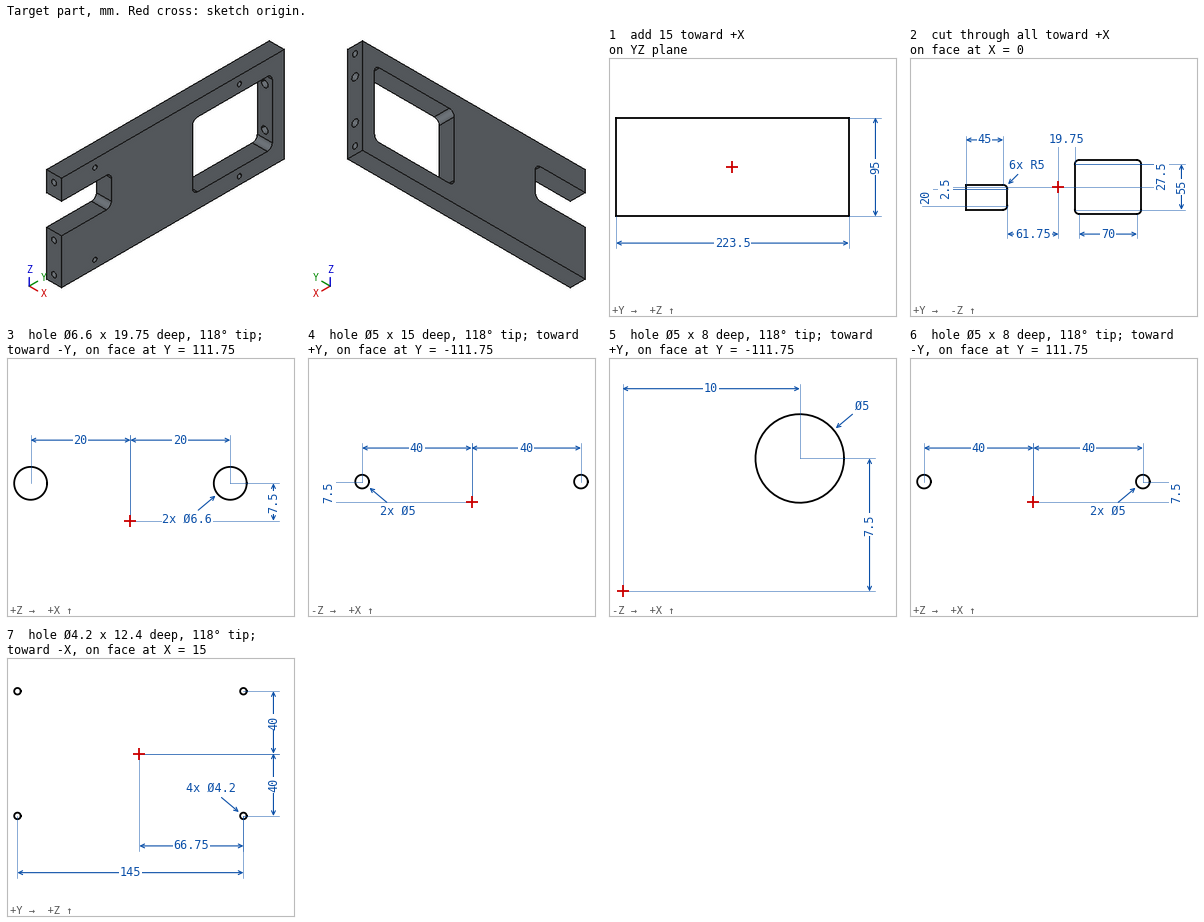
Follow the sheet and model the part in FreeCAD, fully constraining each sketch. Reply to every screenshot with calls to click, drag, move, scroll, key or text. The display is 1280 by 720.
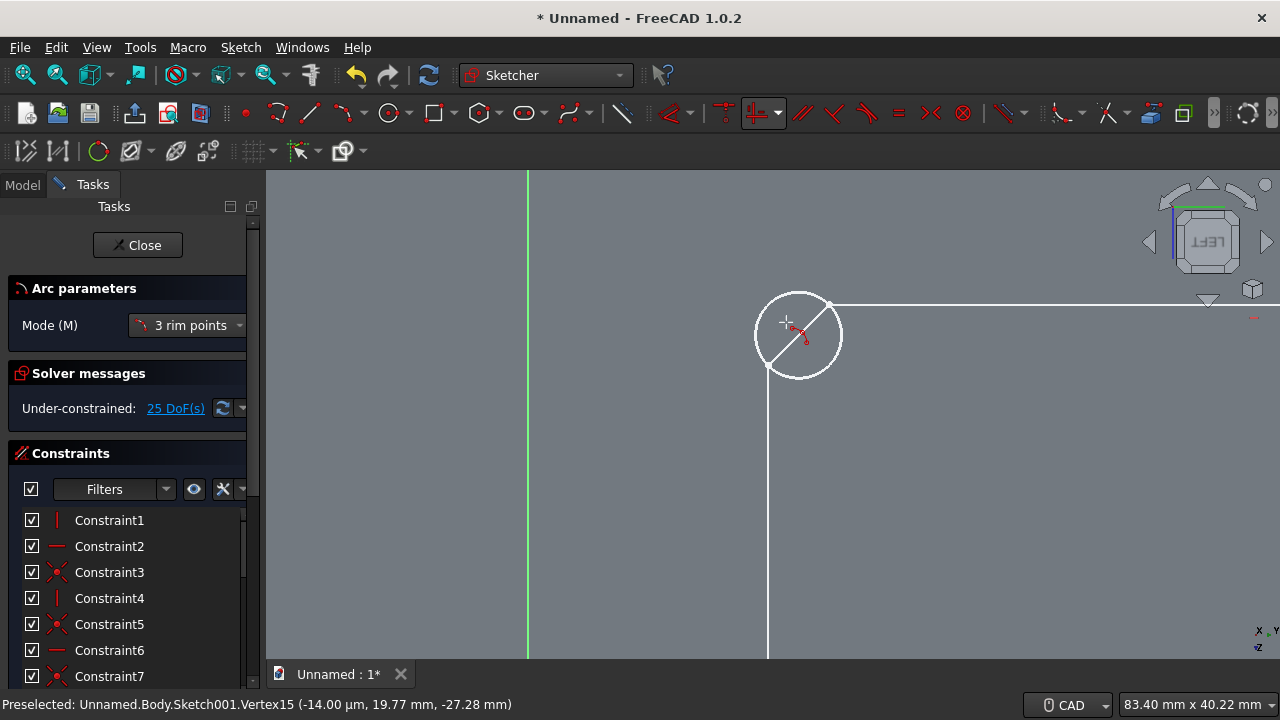
click(786, 320)
key(Escape)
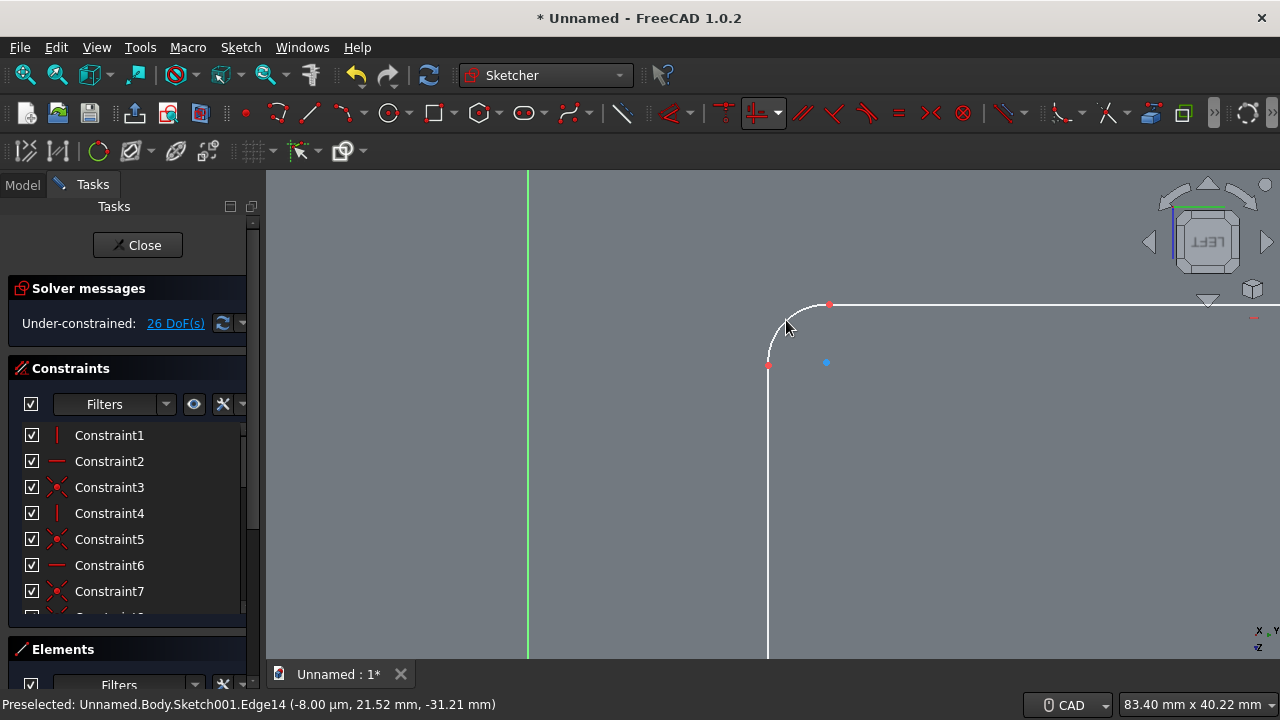
scroll(786, 322, down, 7)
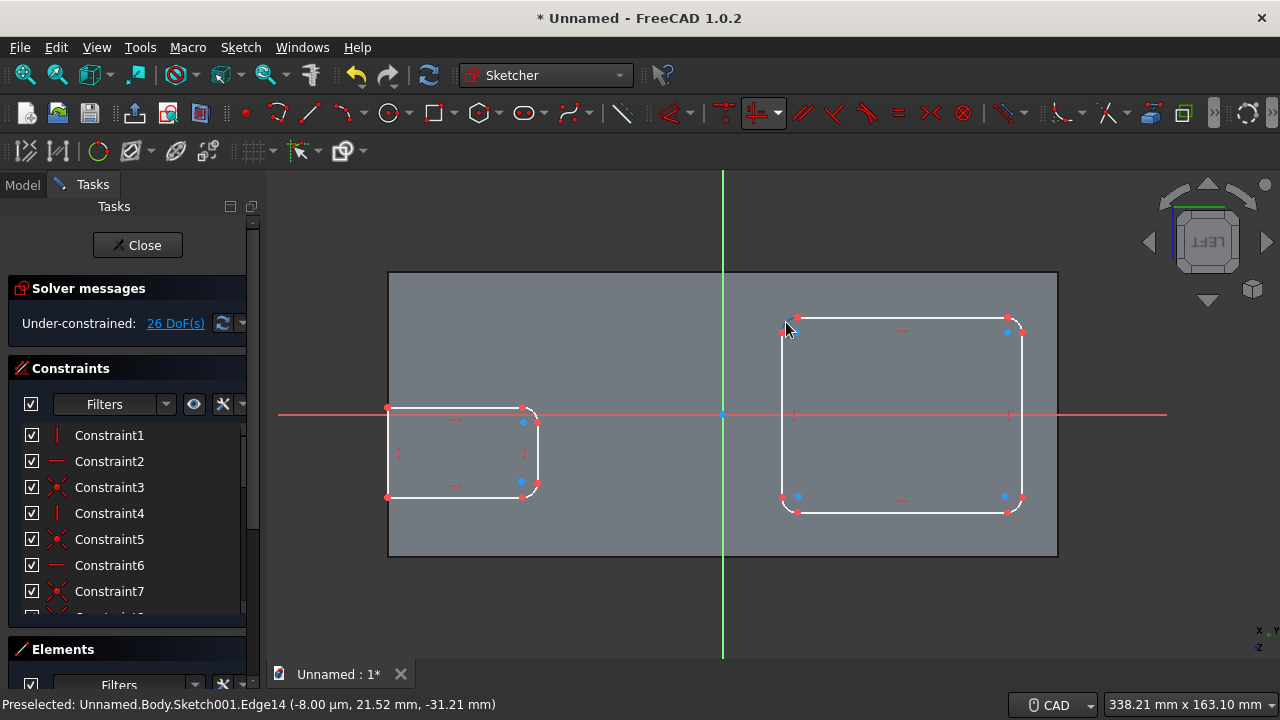
click(538, 465)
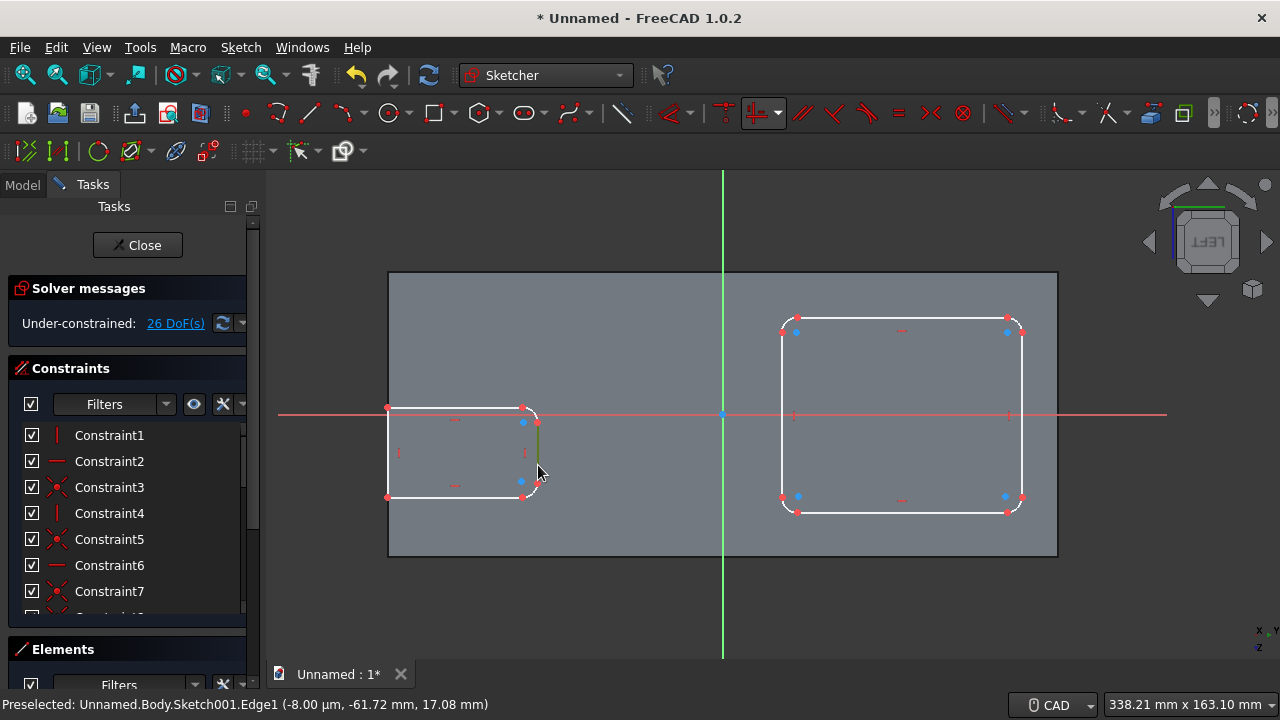
click(533, 412)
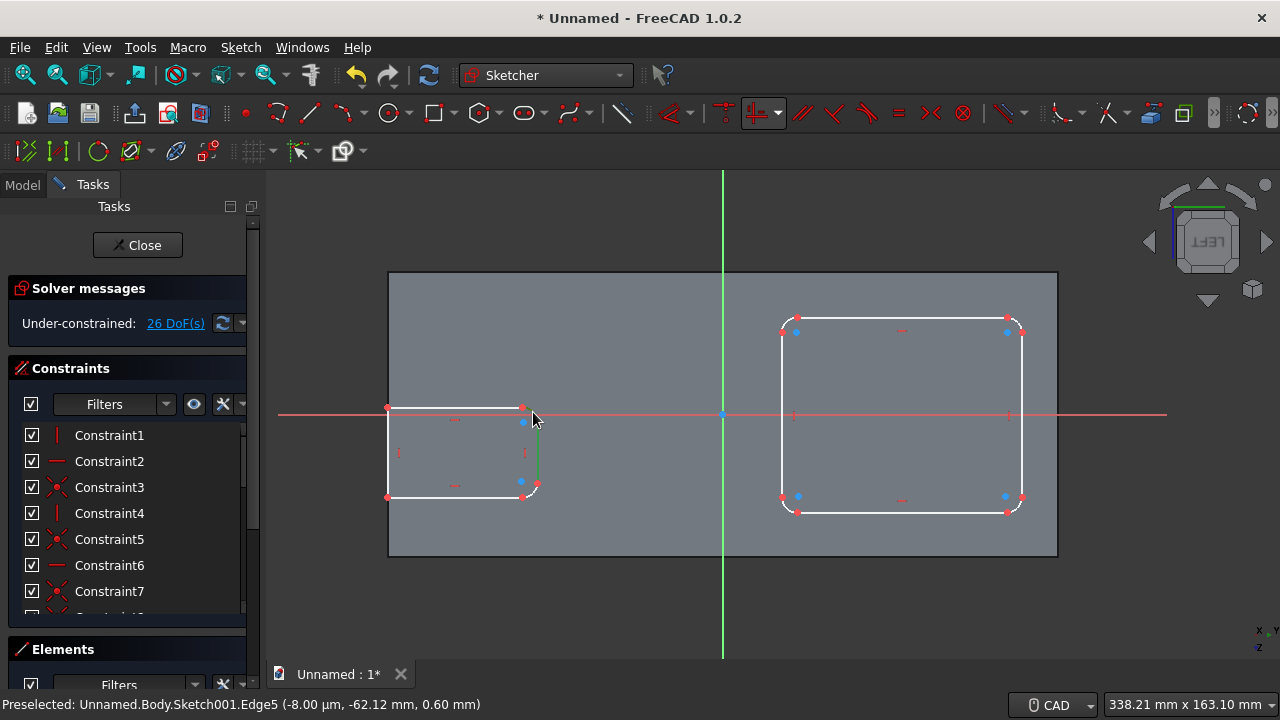
key(t)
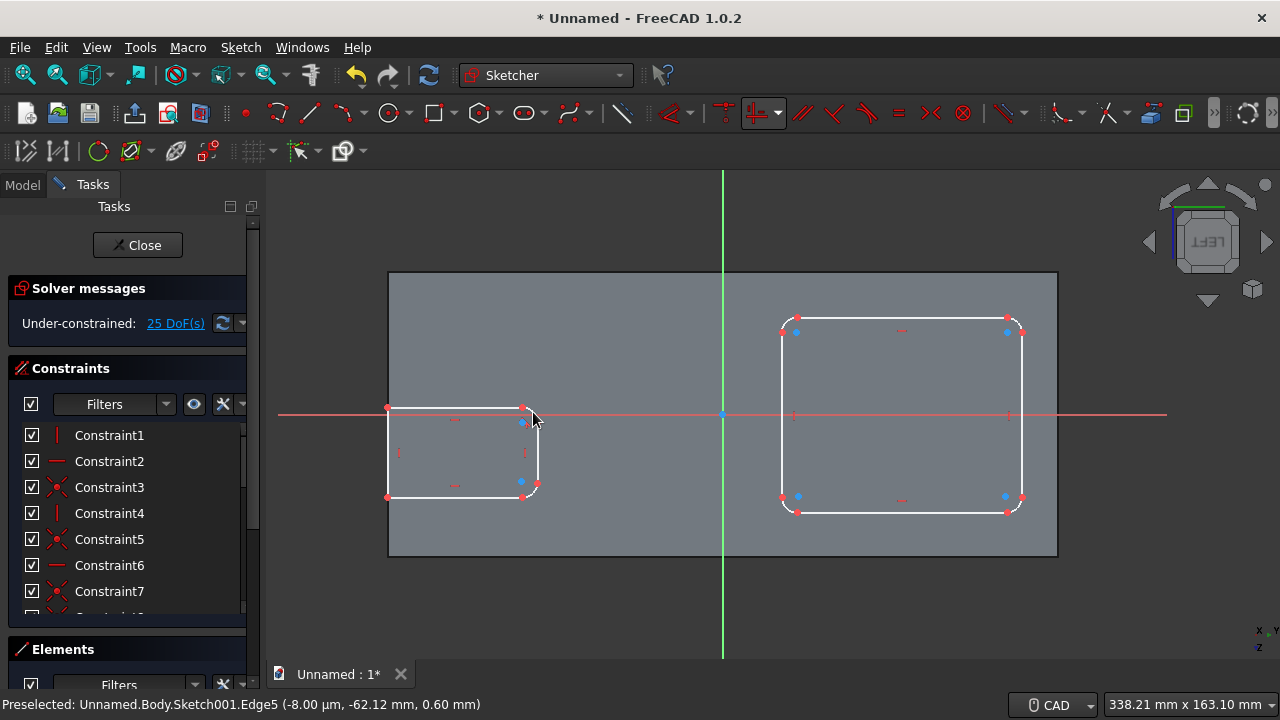
click(538, 465)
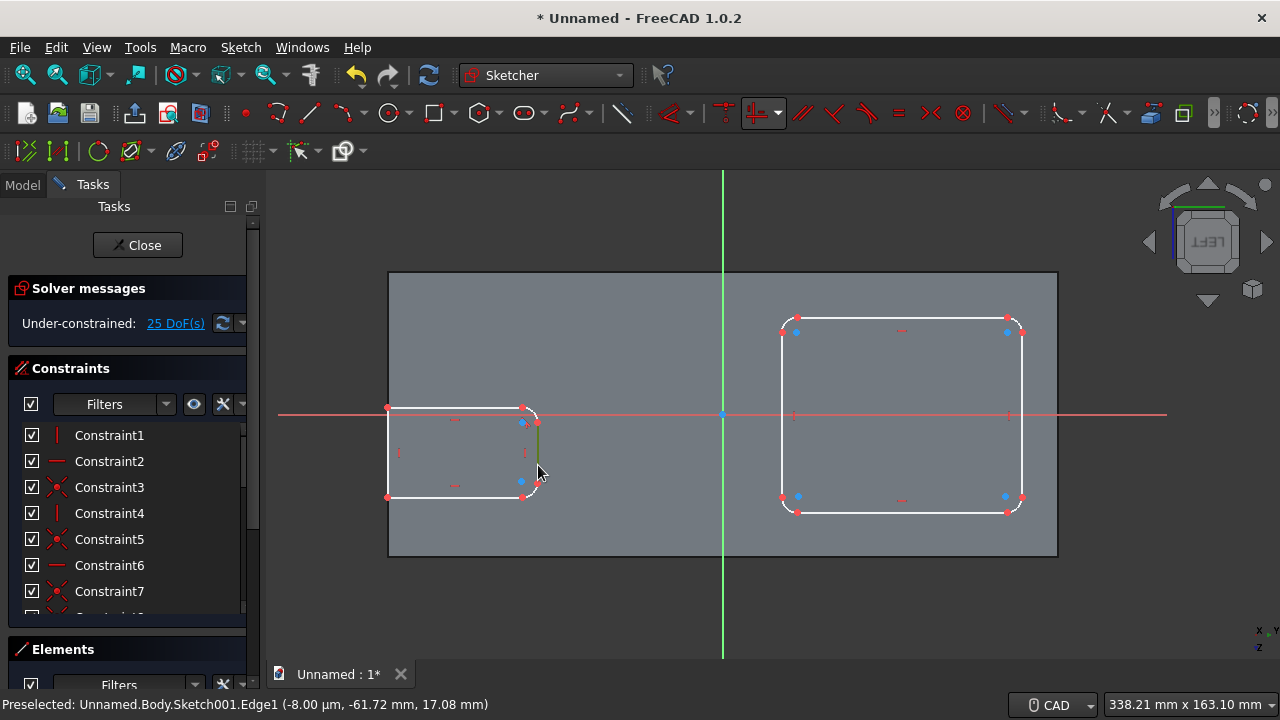
scroll(533, 493, up, 2)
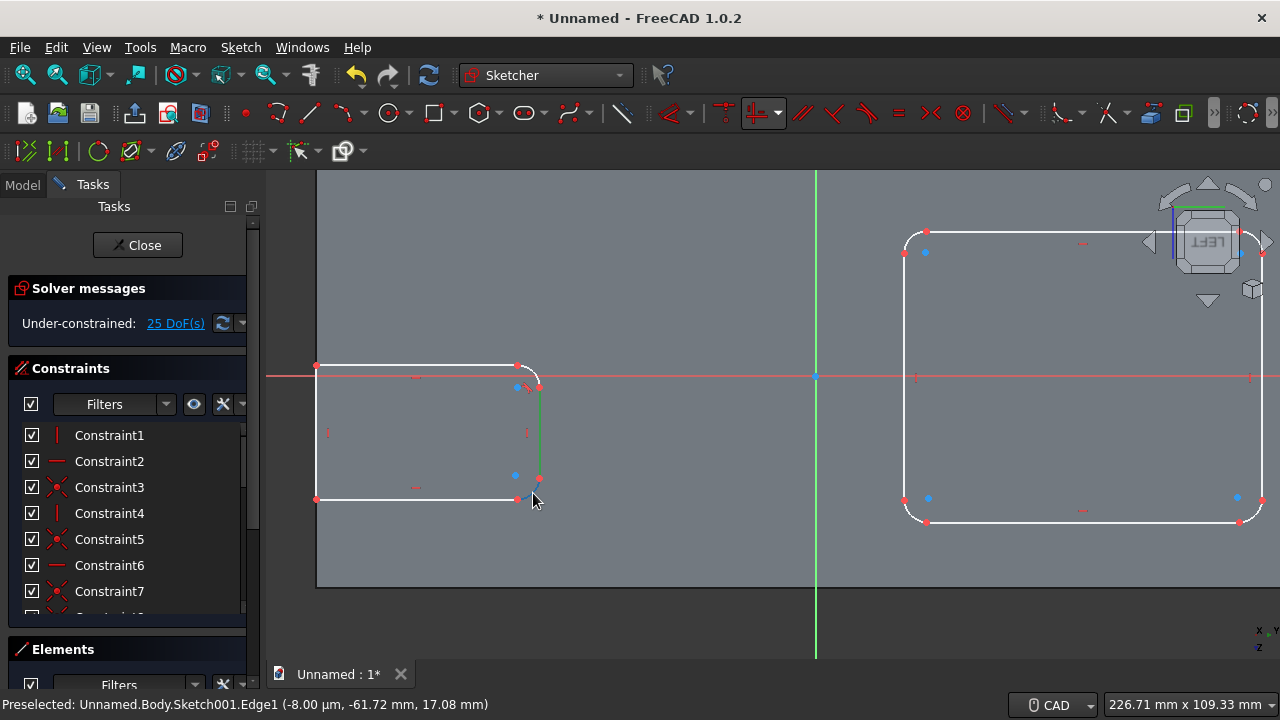
click(533, 493)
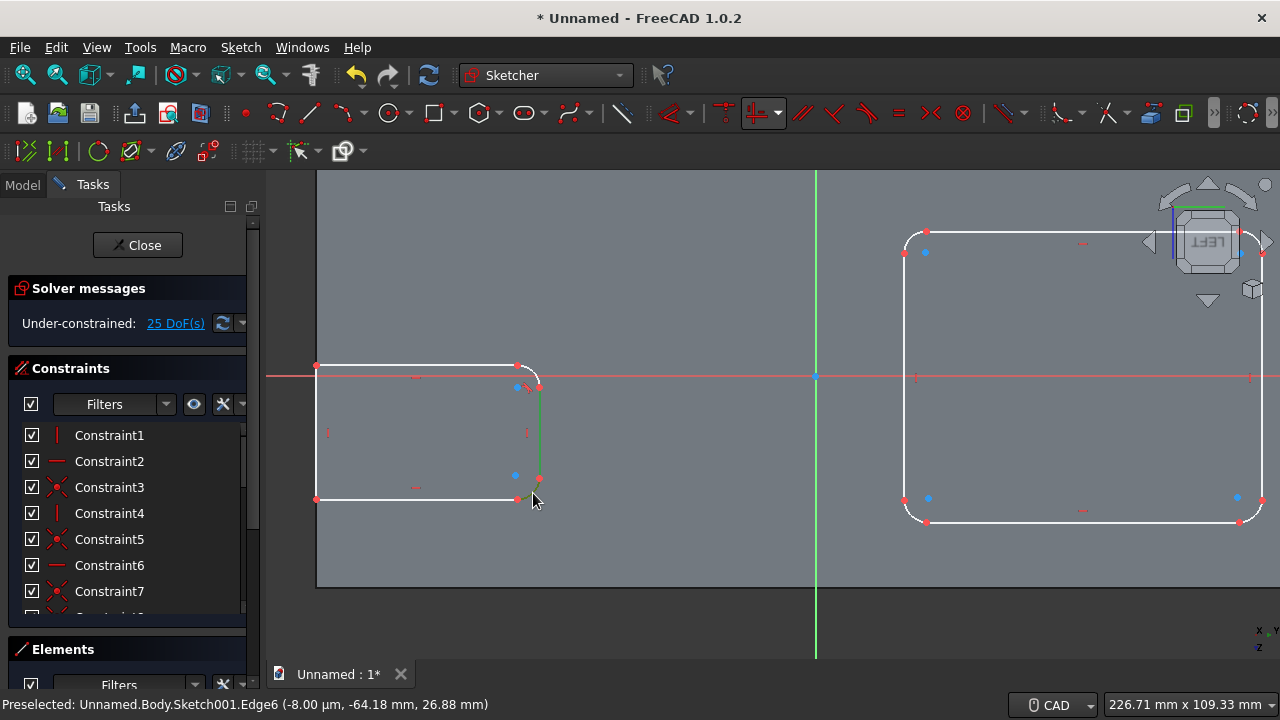
click(868, 114)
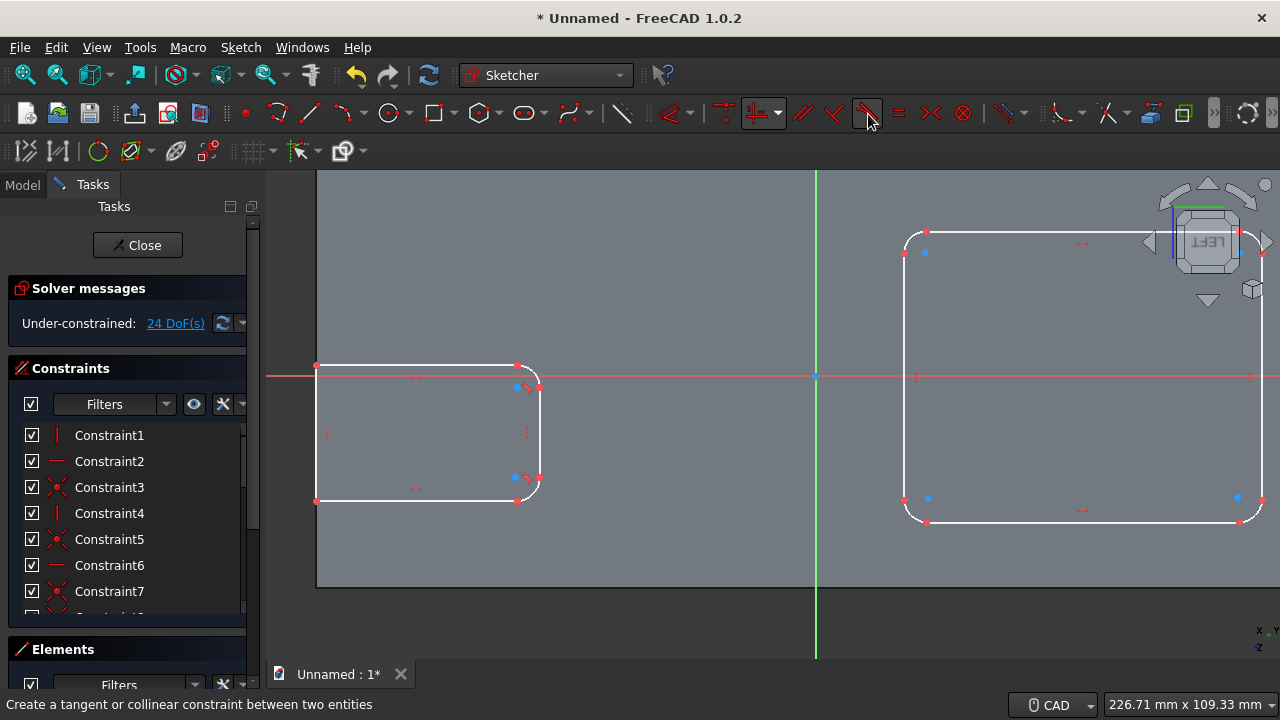
scroll(457, 365, up, 2)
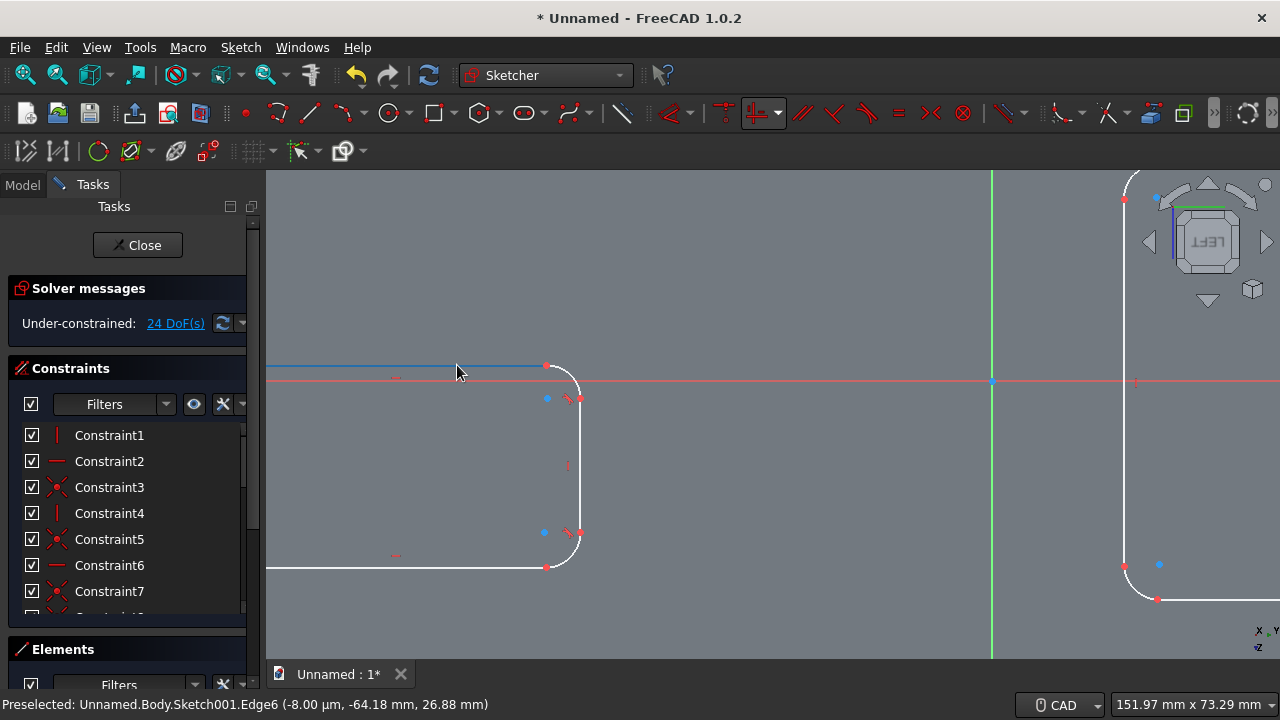
click(457, 366)